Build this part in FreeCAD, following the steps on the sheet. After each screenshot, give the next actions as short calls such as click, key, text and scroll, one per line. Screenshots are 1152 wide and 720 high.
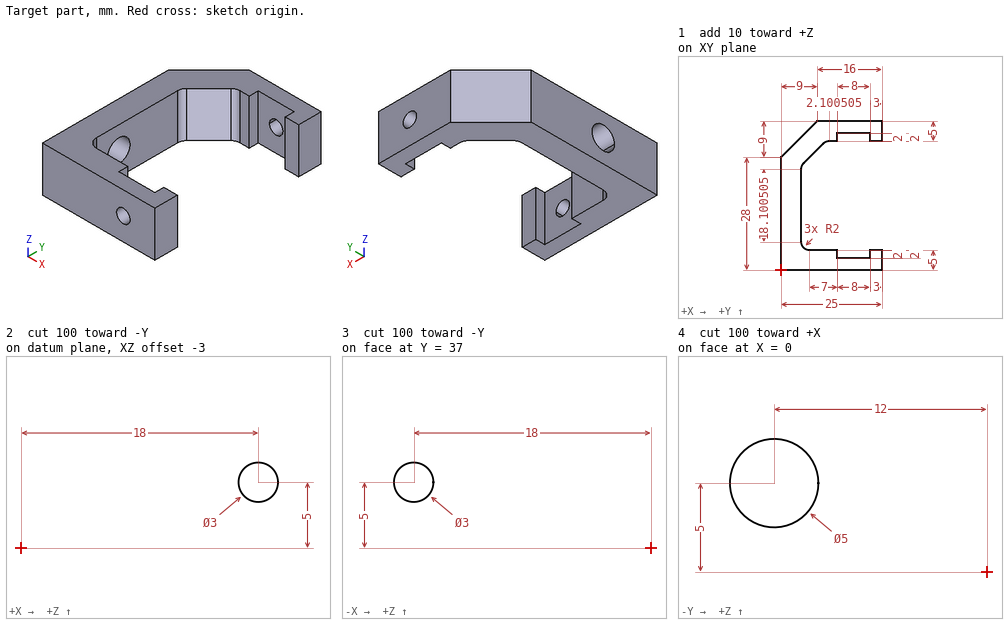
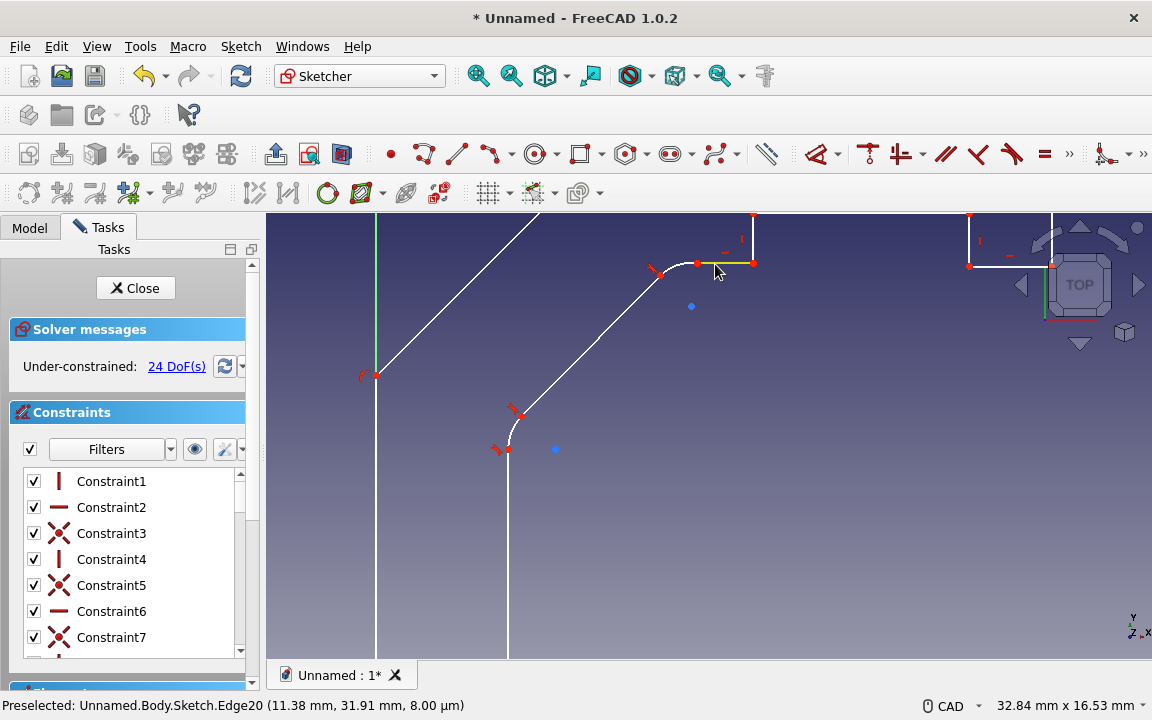
click(714, 263)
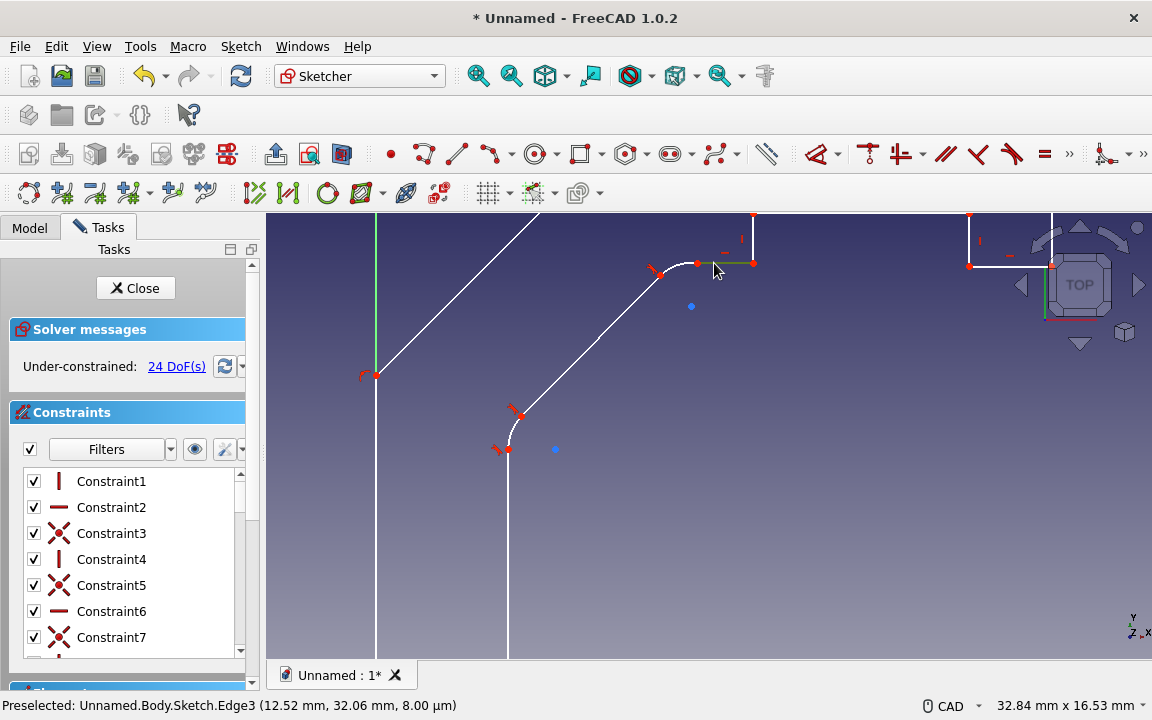
click(686, 263)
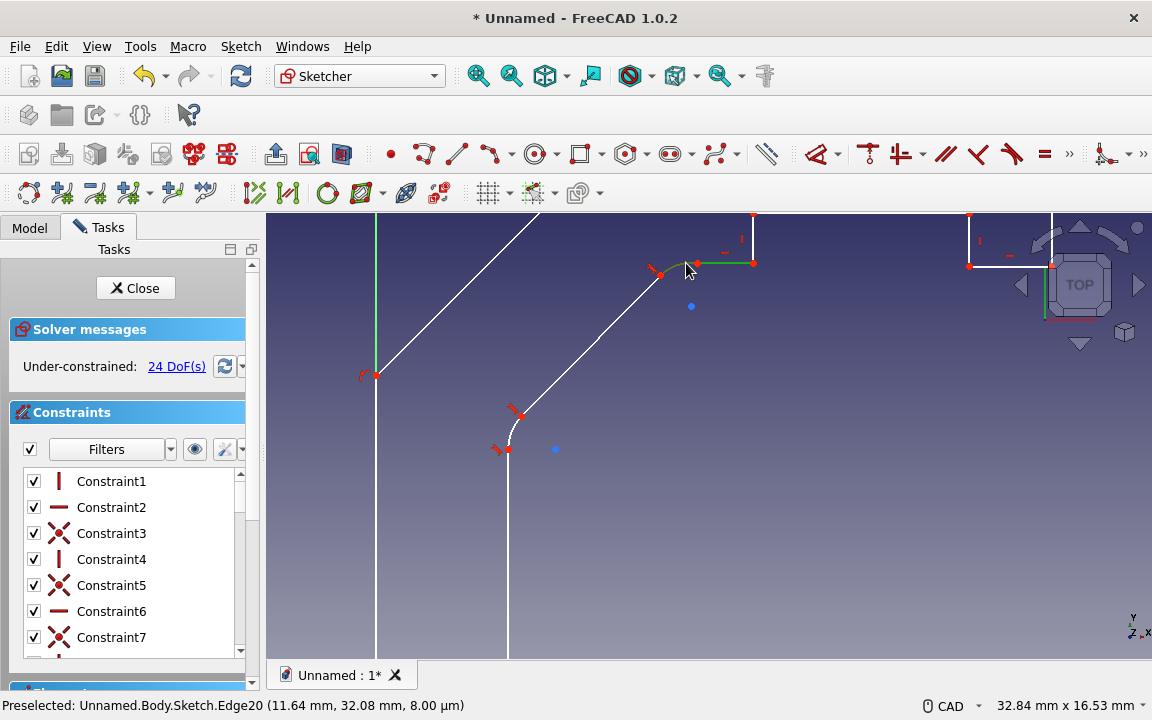
key(t)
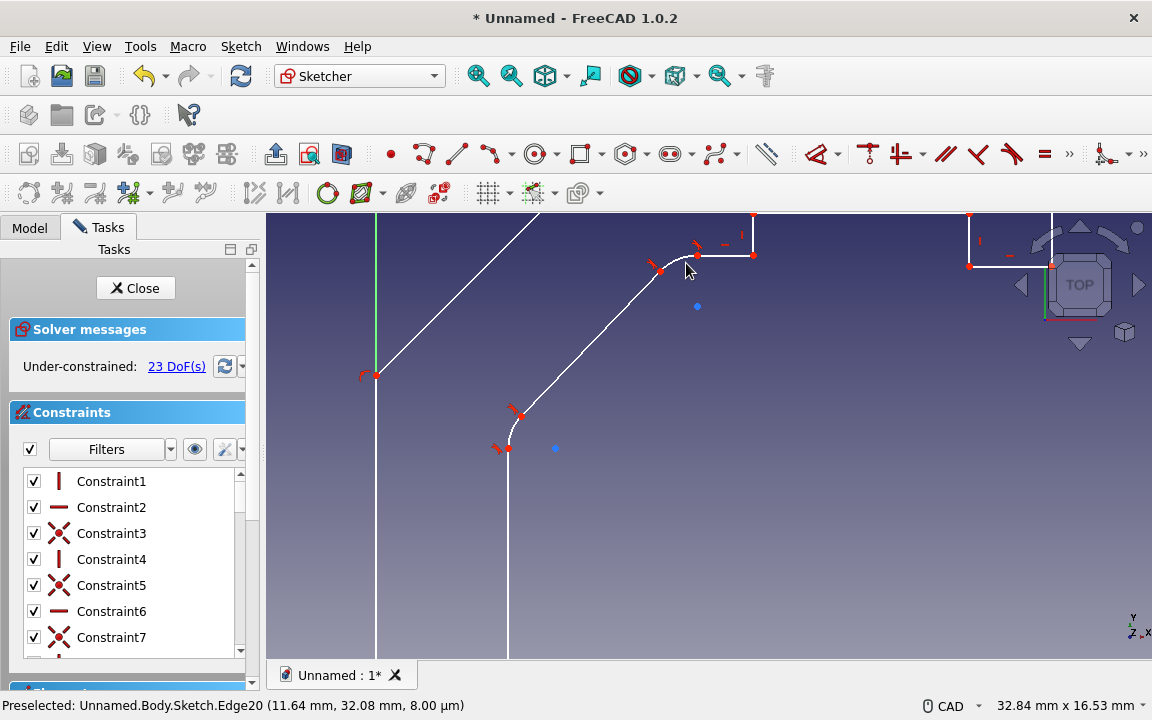
scroll(609, 353, down, 6)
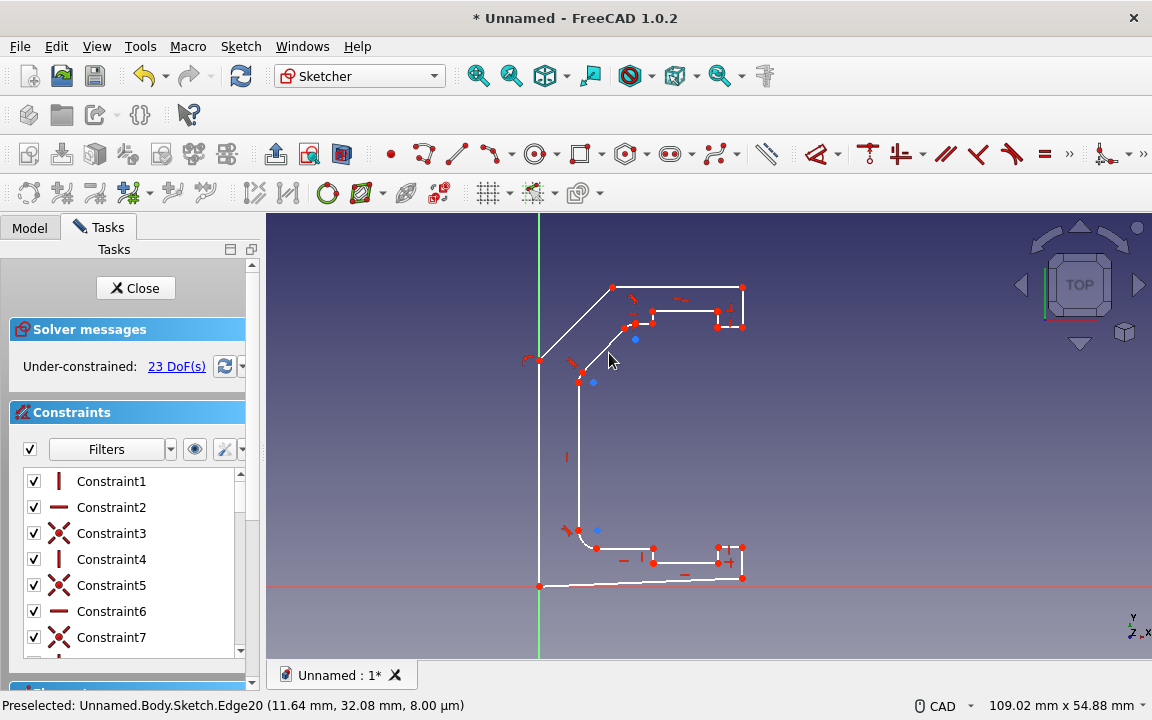
click(636, 549)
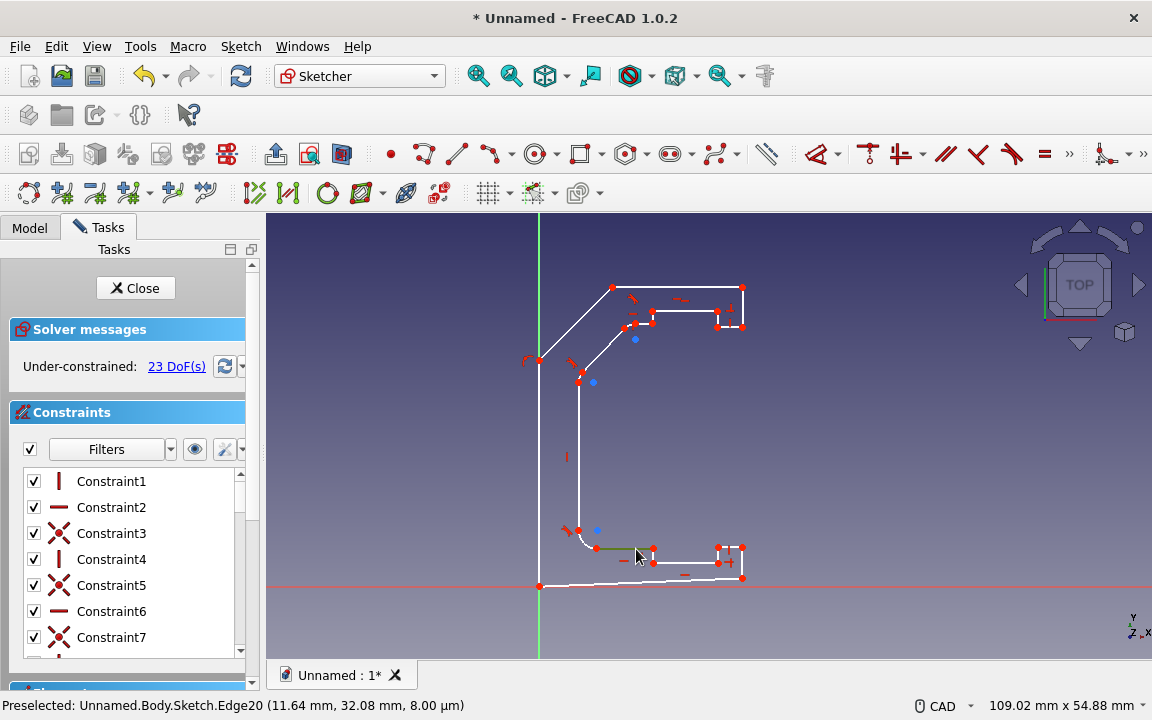
click(584, 543)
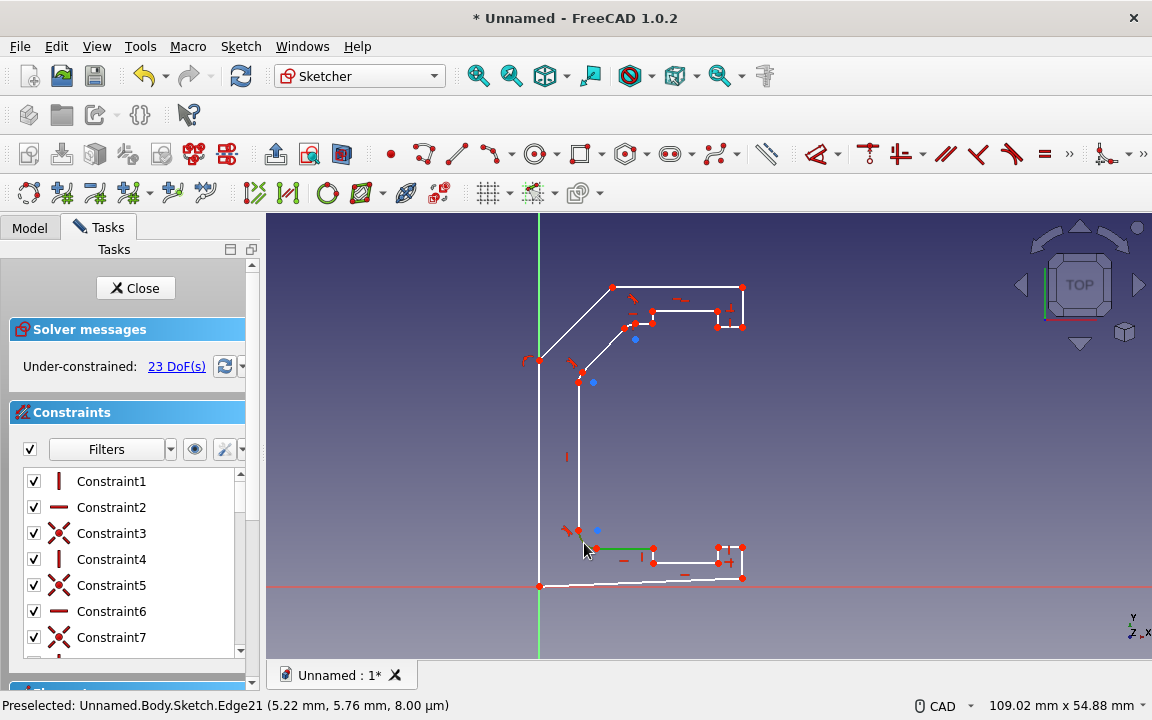
click(1012, 154)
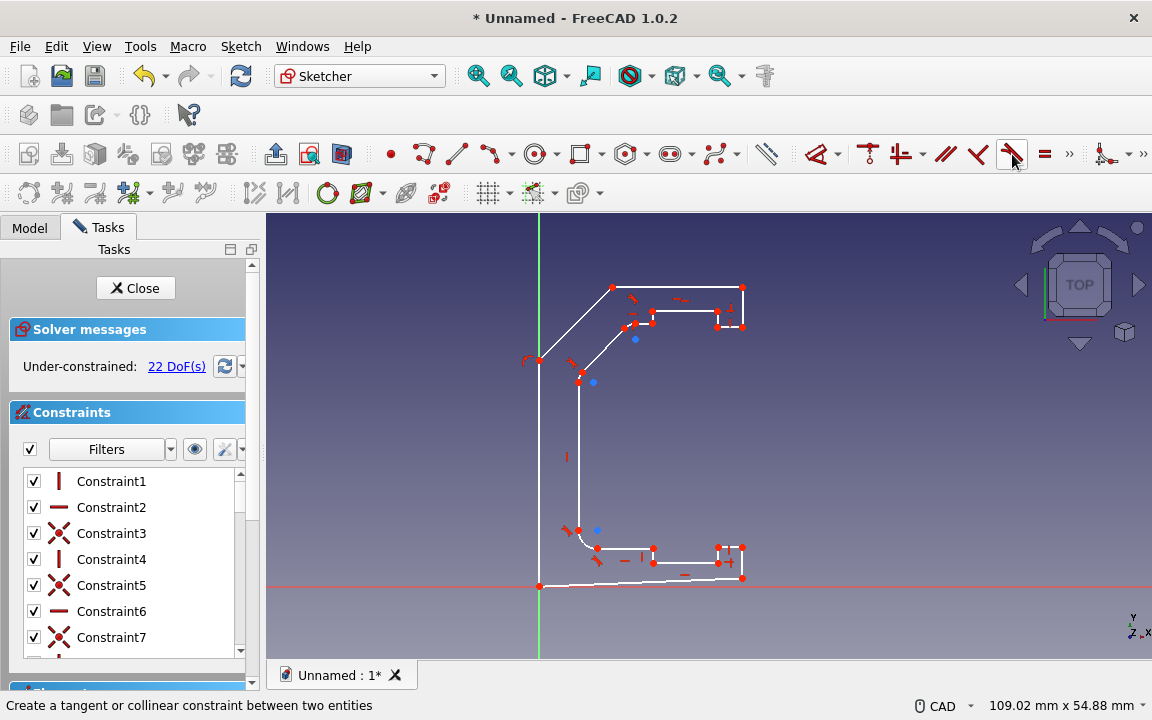
click(600, 584)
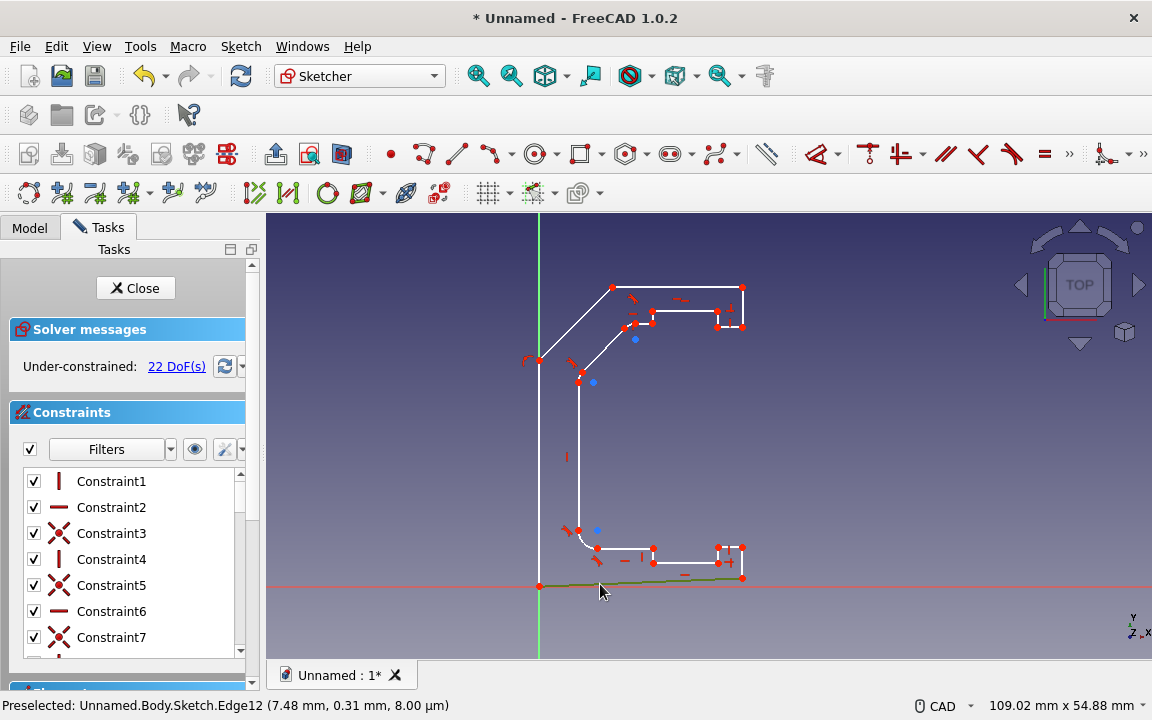
key(h)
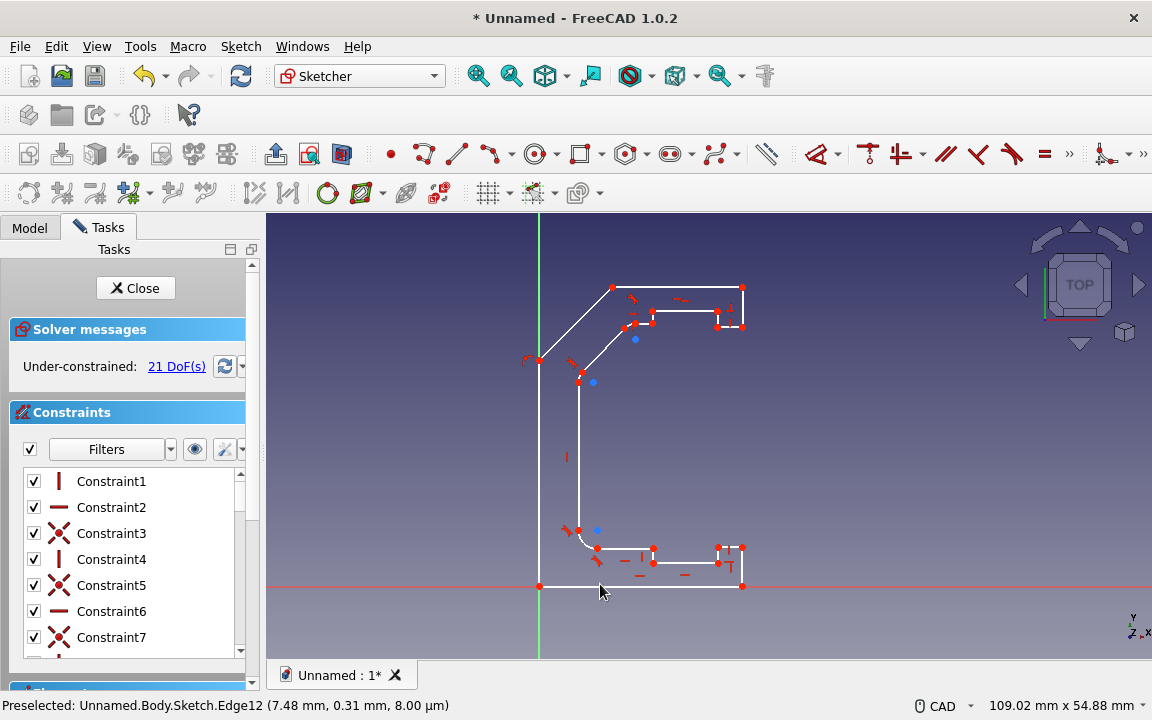
scroll(580, 377, up, 5)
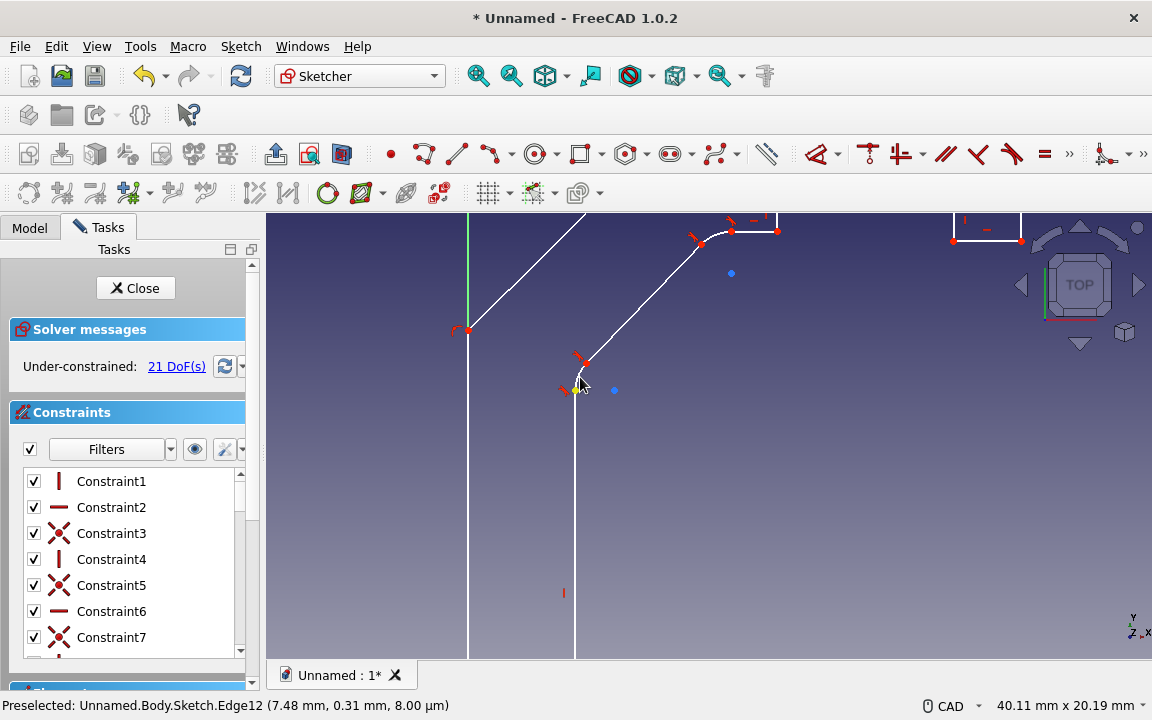
click(578, 376)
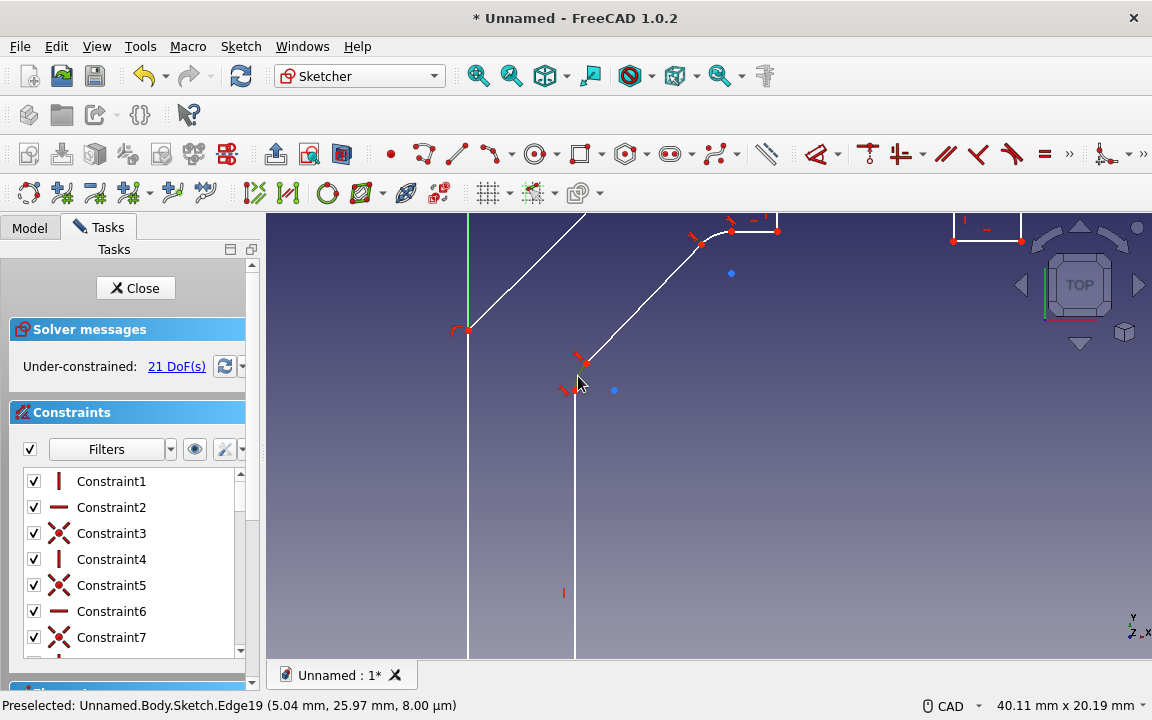
scroll(580, 377, down, 5)